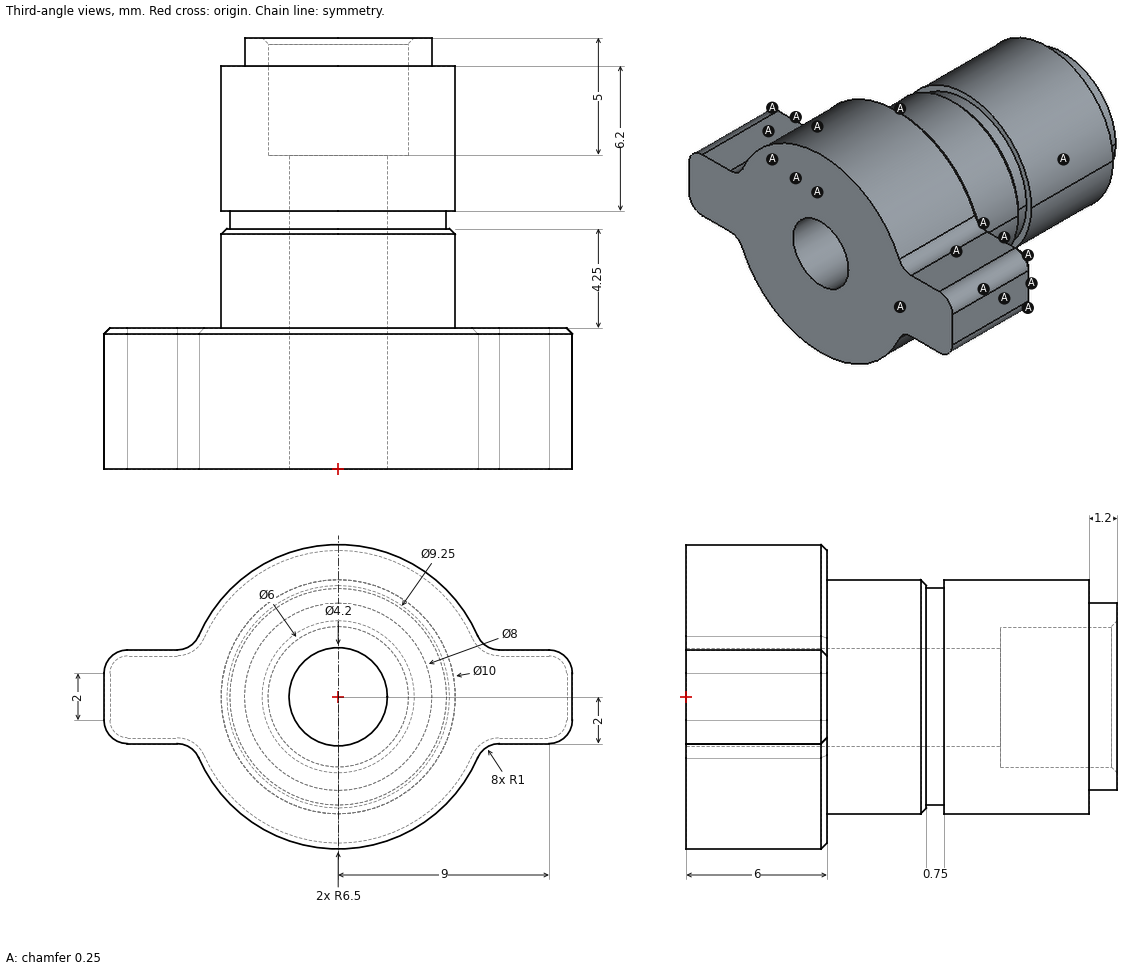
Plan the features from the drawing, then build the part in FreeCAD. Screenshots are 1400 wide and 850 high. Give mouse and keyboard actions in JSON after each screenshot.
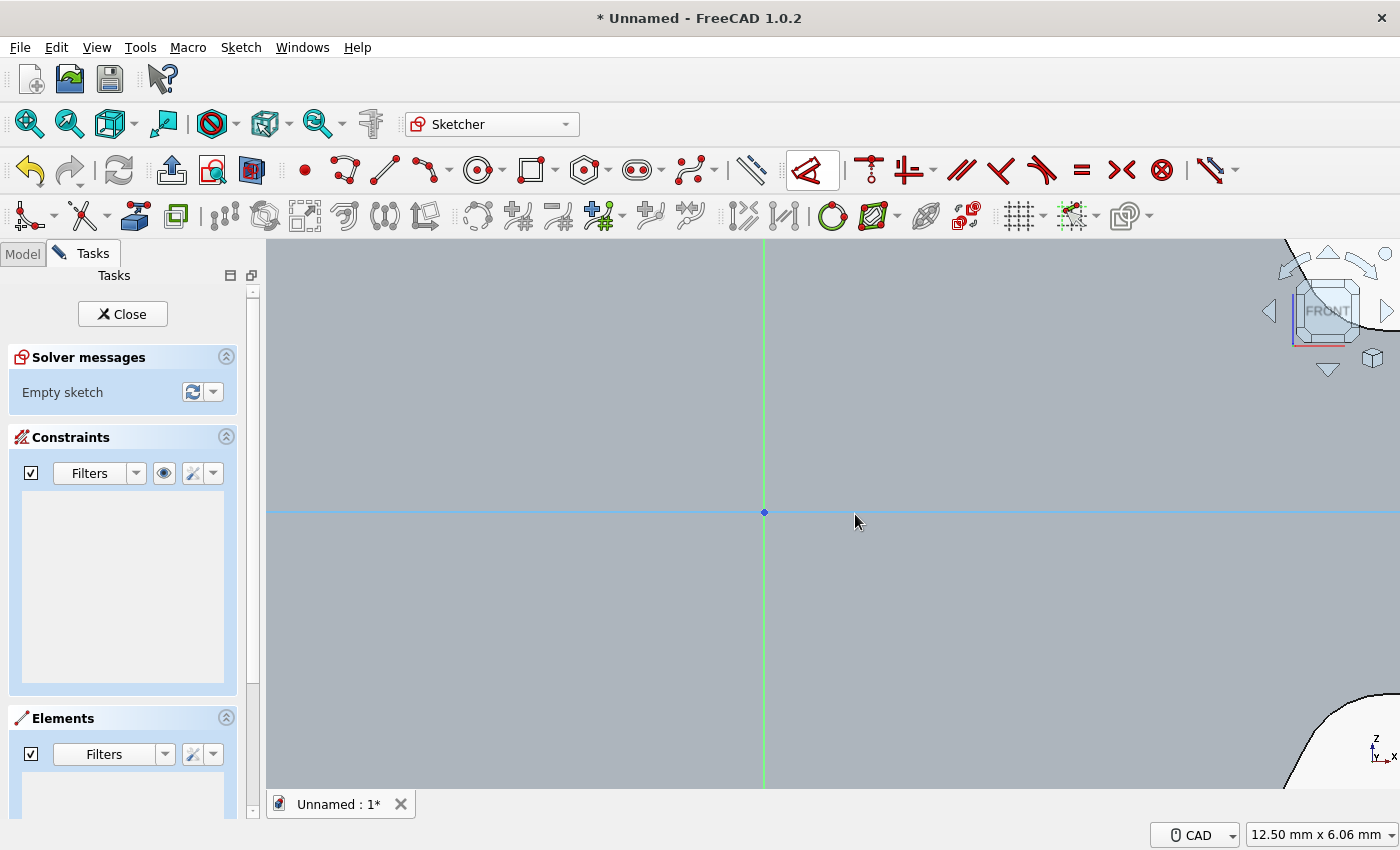
{"action": "left_click", "coordinate": [478, 170]}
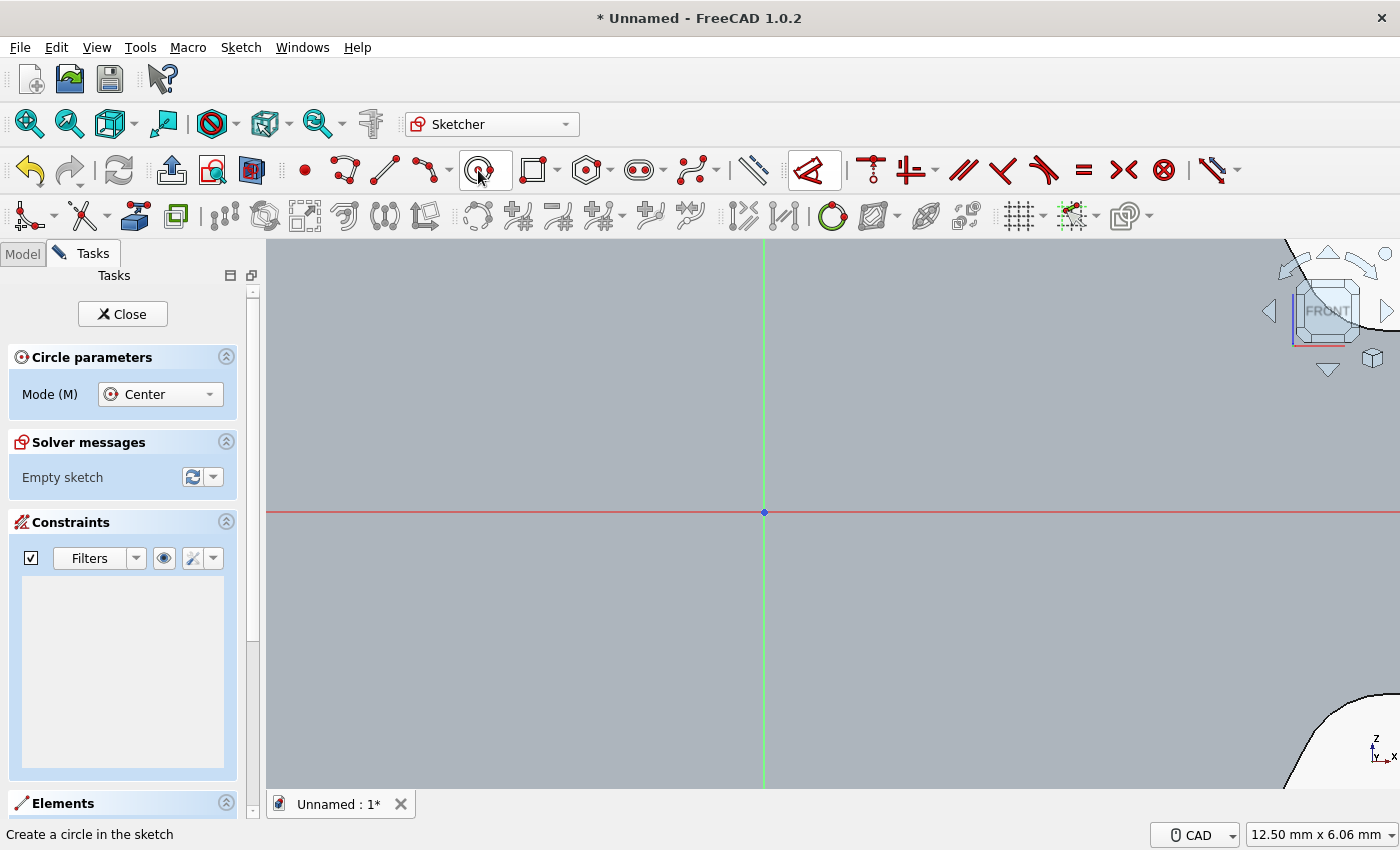
{"action": "left_click", "coordinate": [764, 512]}
{"action": "mouse_move", "coordinate": [899, 378]}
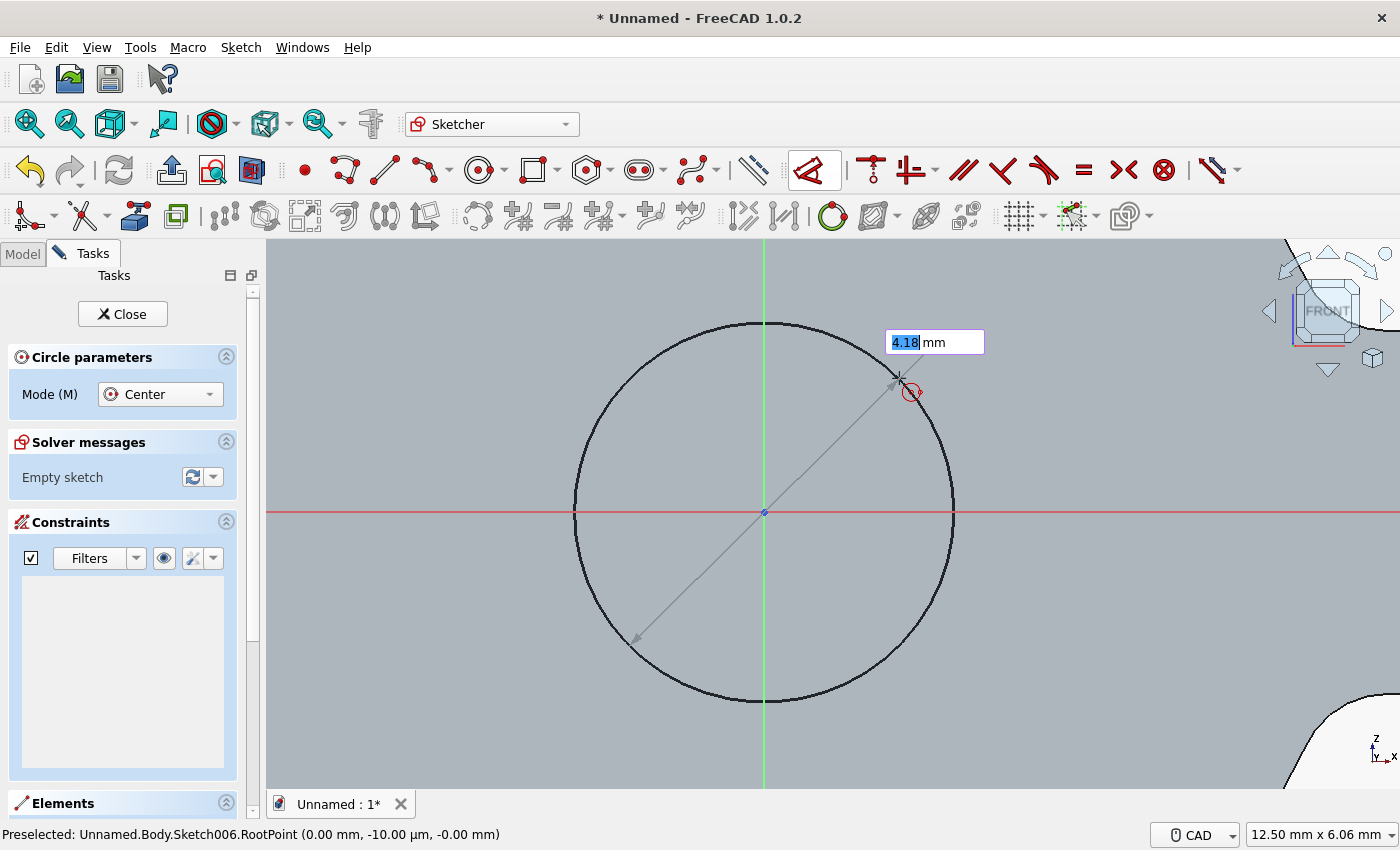
{"action": "type", "text": "4.2"}
{"action": "key", "text": "Return"}
{"action": "key", "text": "Escape"}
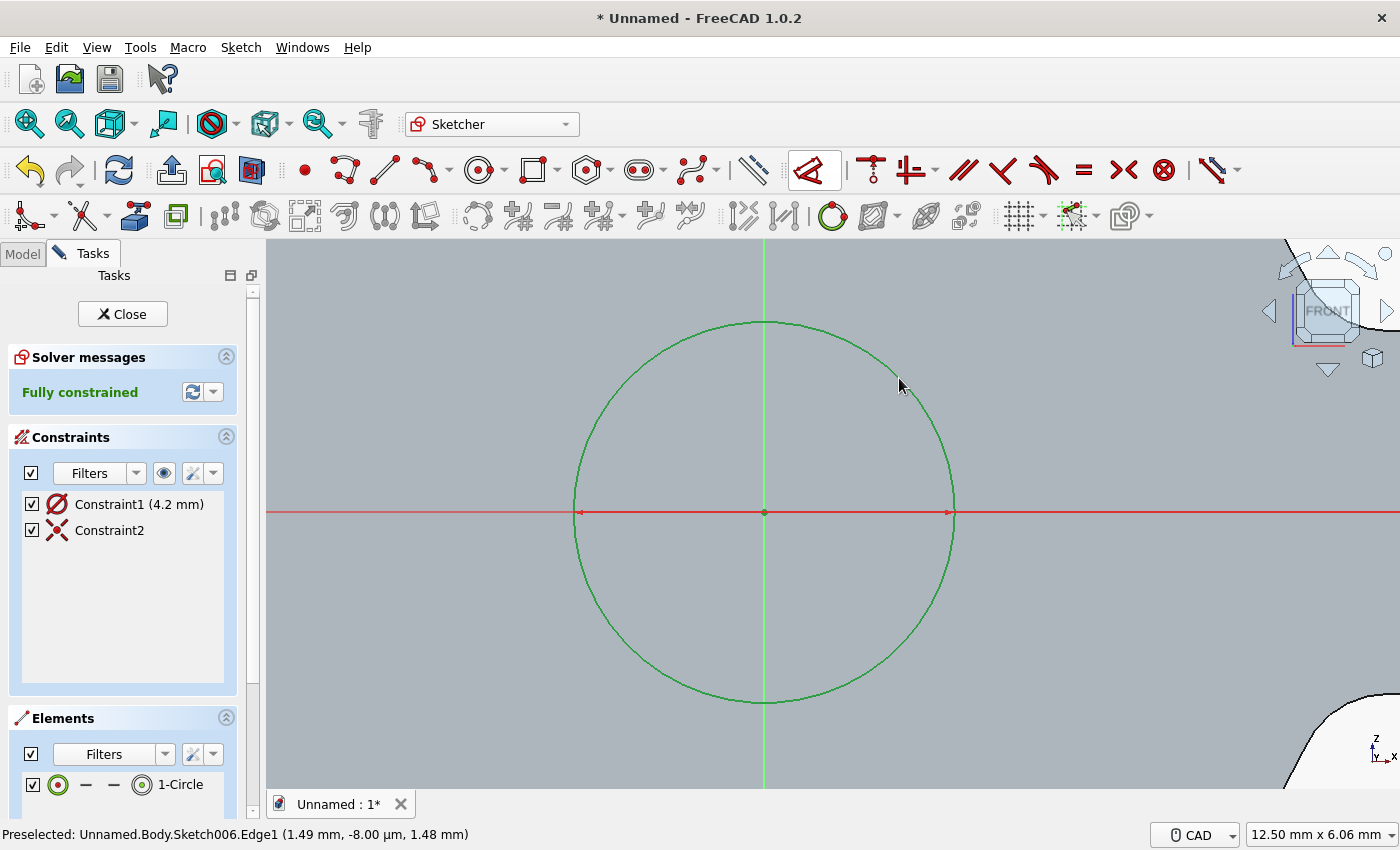
{"action": "left_click", "coordinate": [123, 314]}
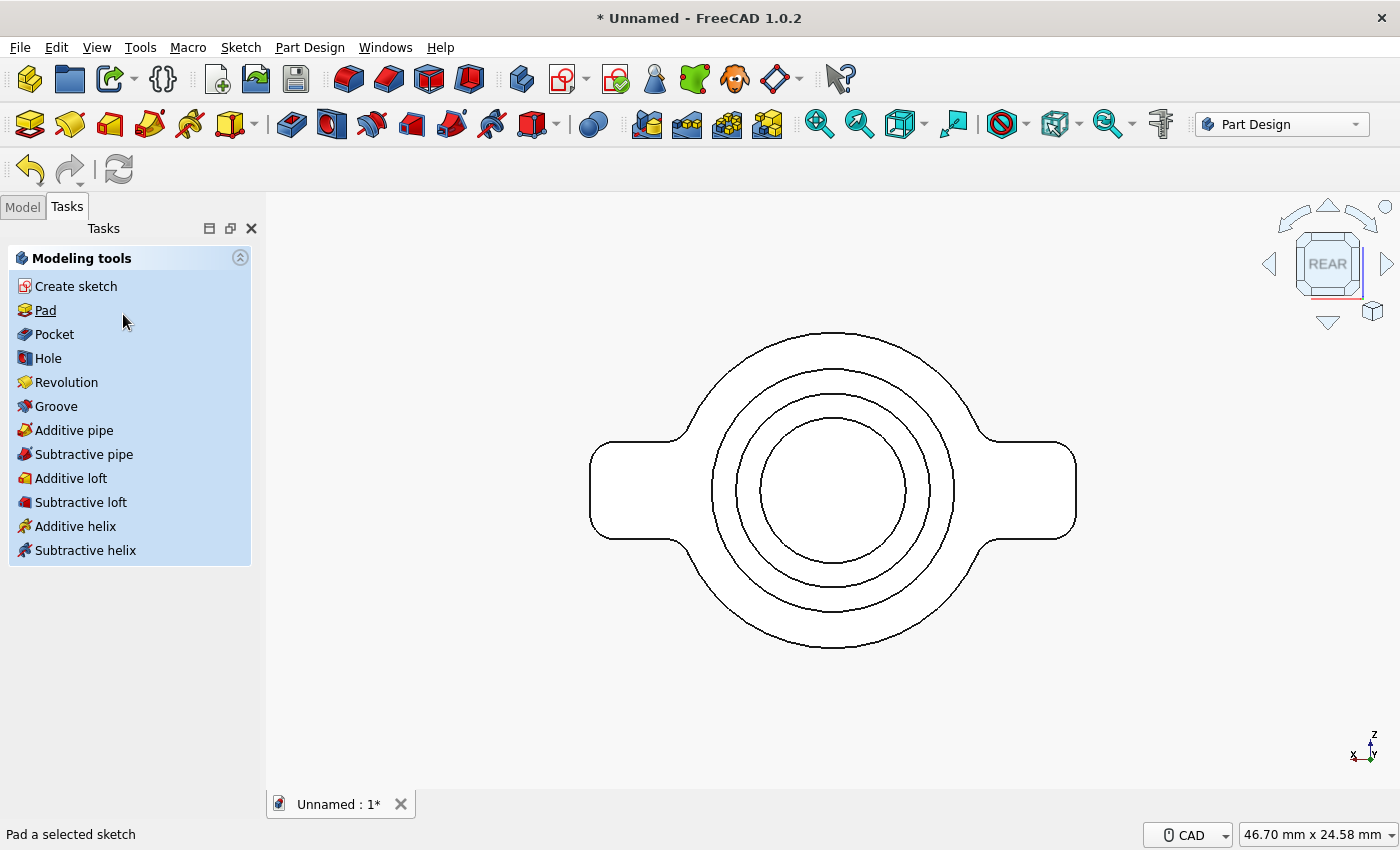
{"action": "left_click", "coordinate": [292, 124]}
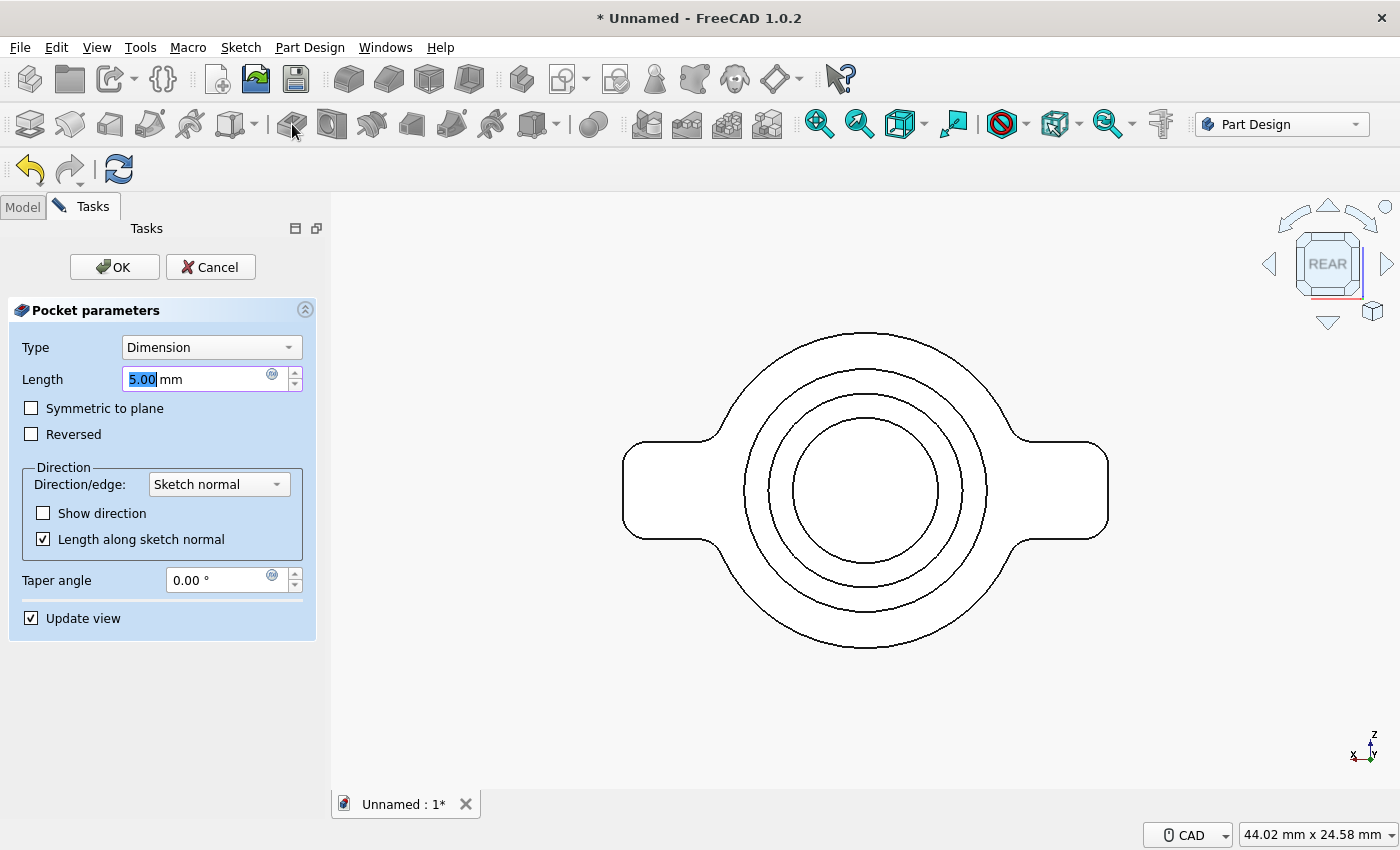
{"action": "left_click", "coordinate": [212, 348]}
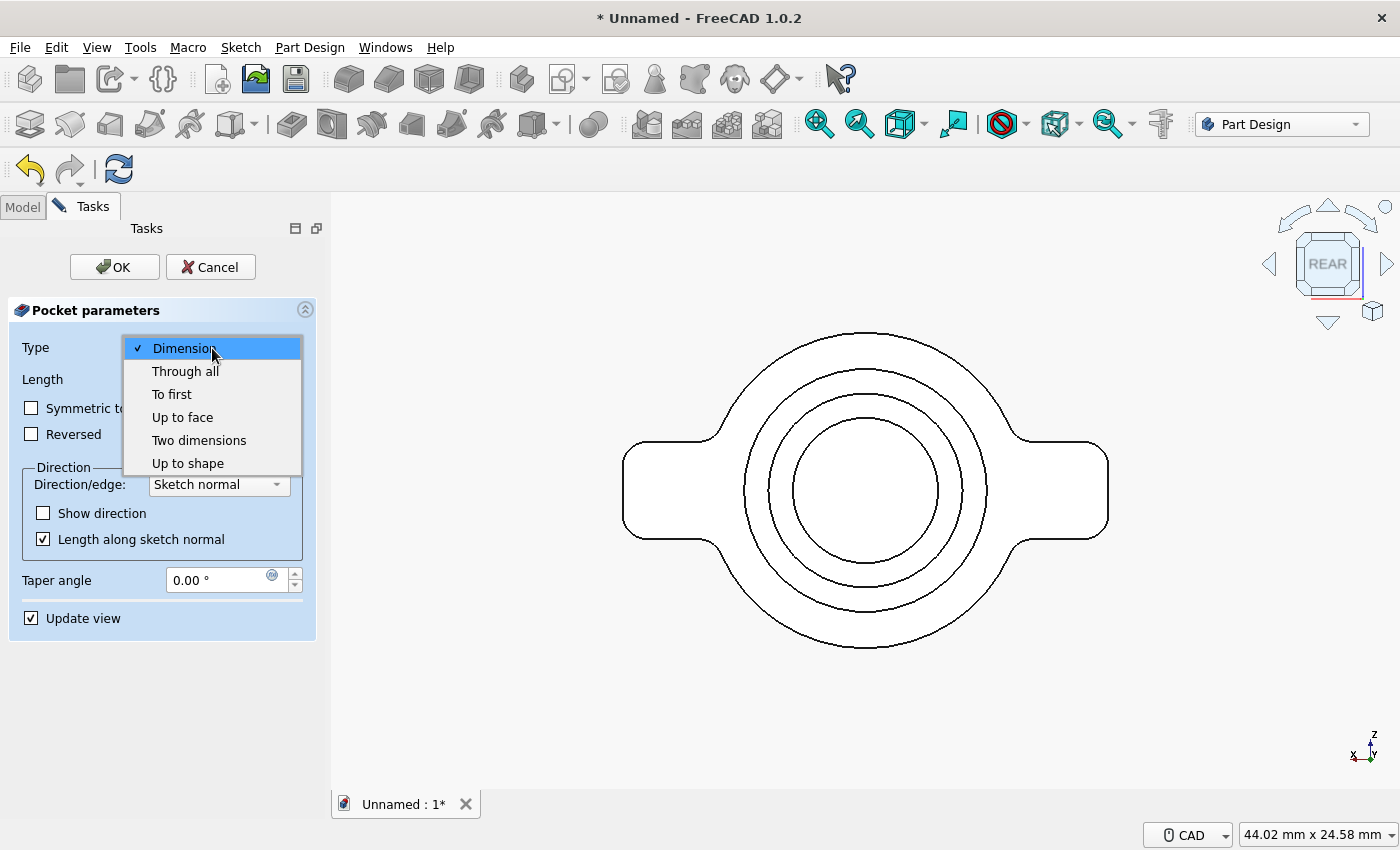
{"action": "left_click", "coordinate": [212, 372]}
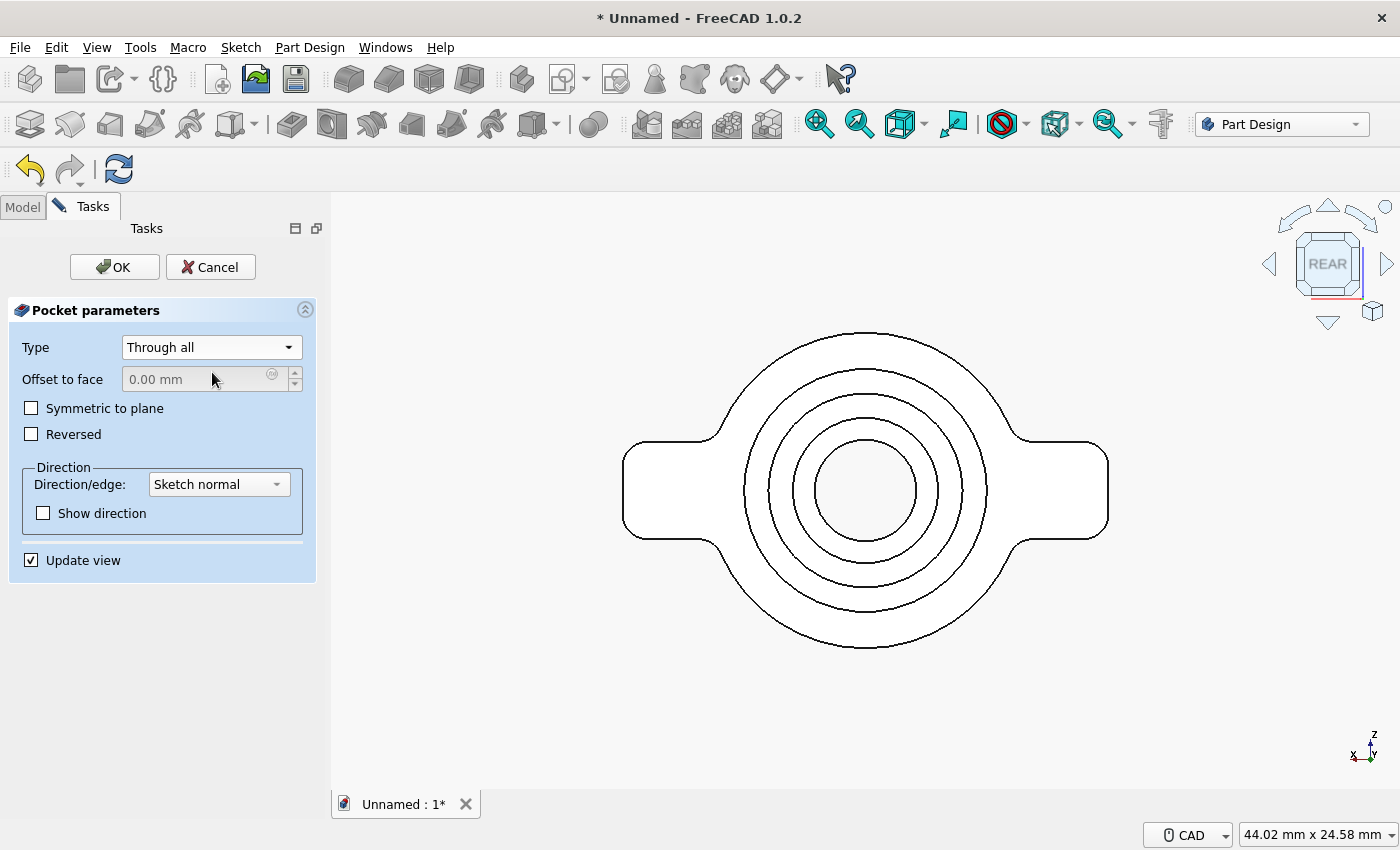
{"action": "left_click", "coordinate": [115, 267]}